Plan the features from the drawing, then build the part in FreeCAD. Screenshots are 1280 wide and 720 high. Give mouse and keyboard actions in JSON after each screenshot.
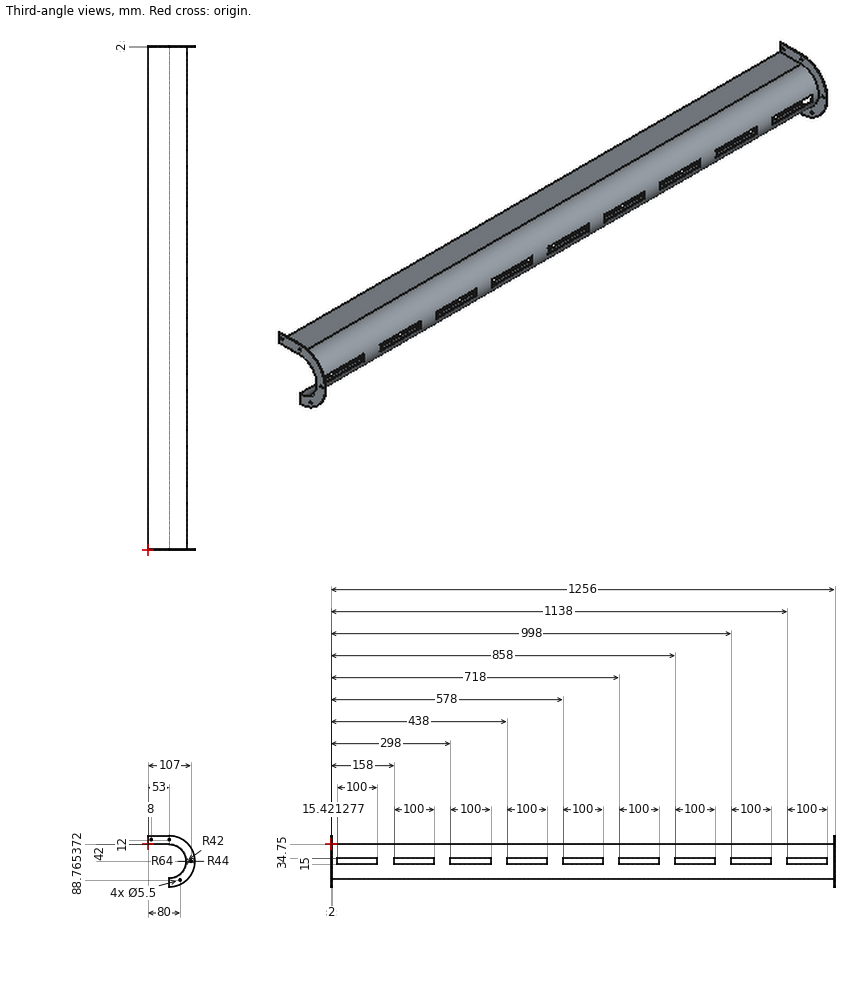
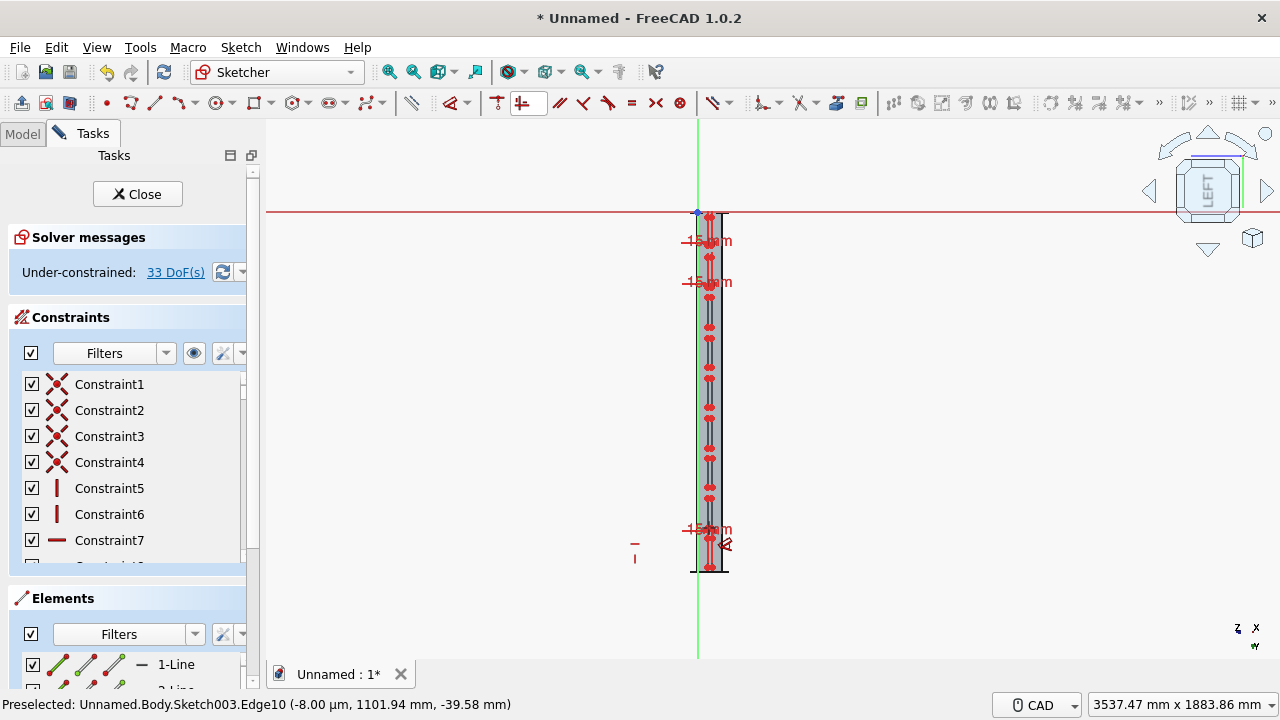
{"action": "scroll", "coordinate": [709, 327], "scroll_direction": "up", "scroll_amount": 12}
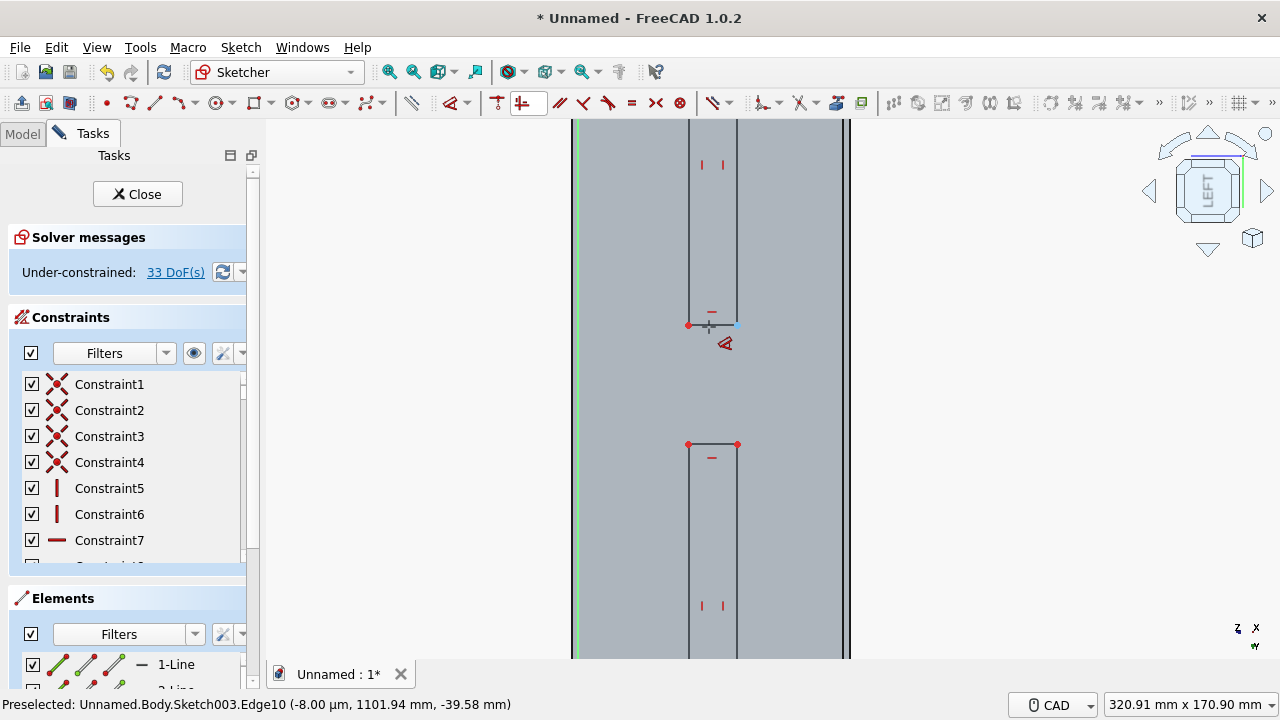
{"action": "left_click", "coordinate": [703, 325]}
{"action": "left_click", "coordinate": [713, 291]}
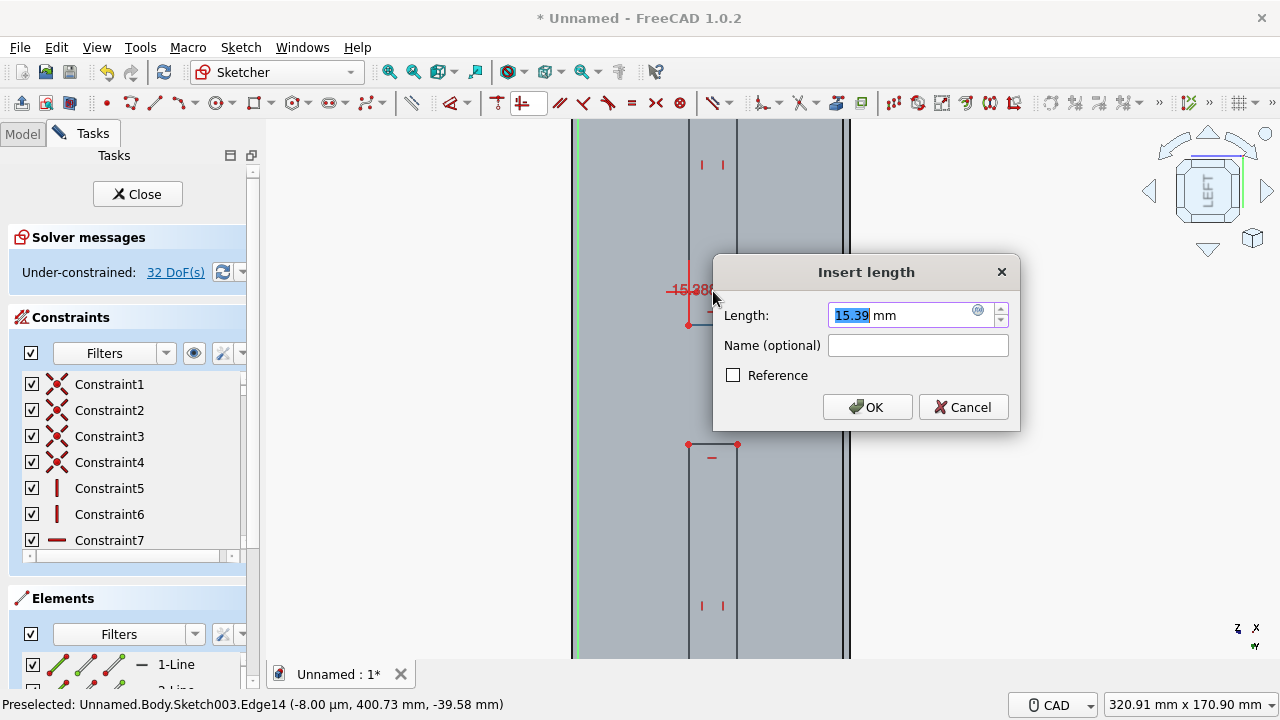
{"action": "type", "text": "15"}
{"action": "key", "text": "Return"}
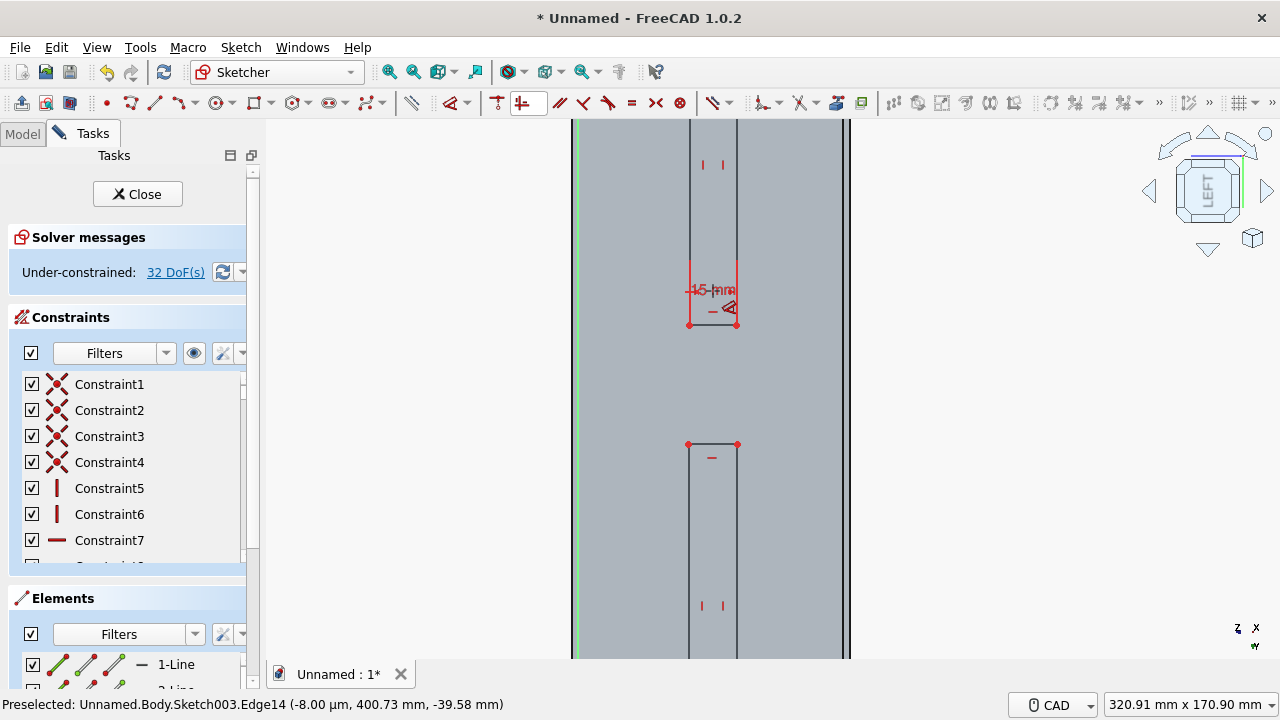
{"action": "scroll", "coordinate": [709, 327], "scroll_direction": "down", "scroll_amount": 12}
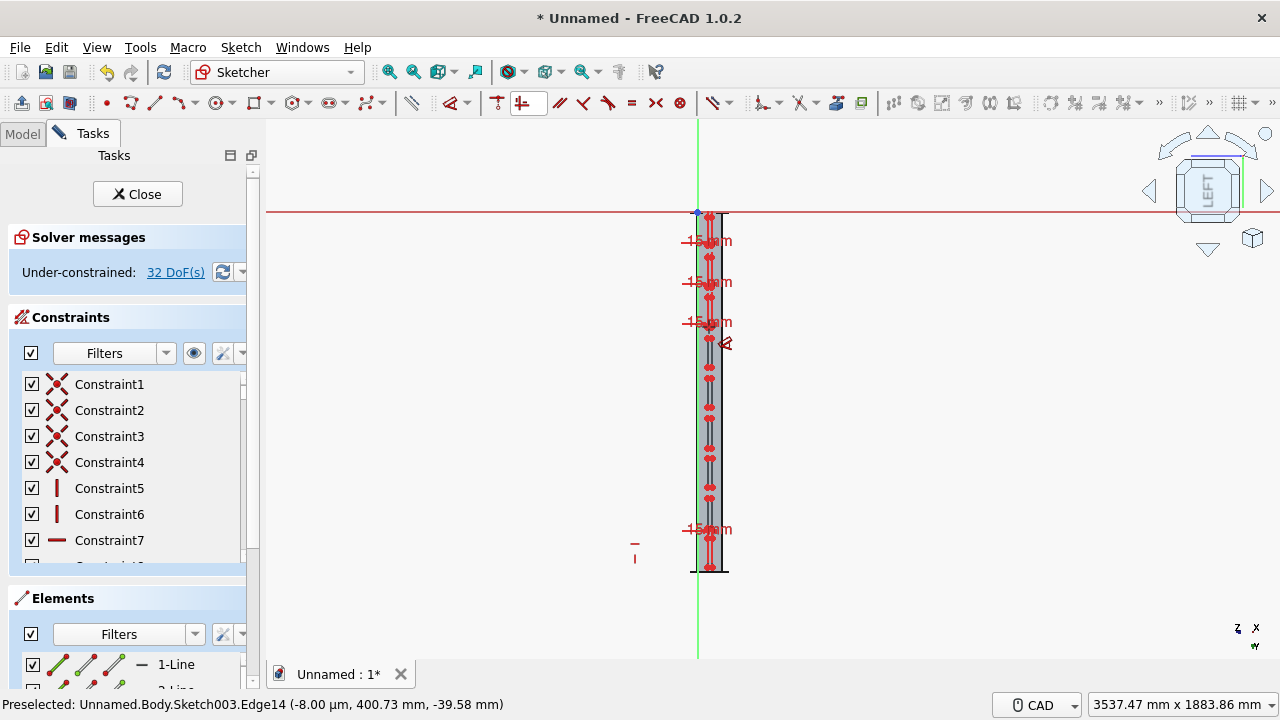
{"action": "scroll", "coordinate": [709, 367], "scroll_direction": "up", "scroll_amount": 12}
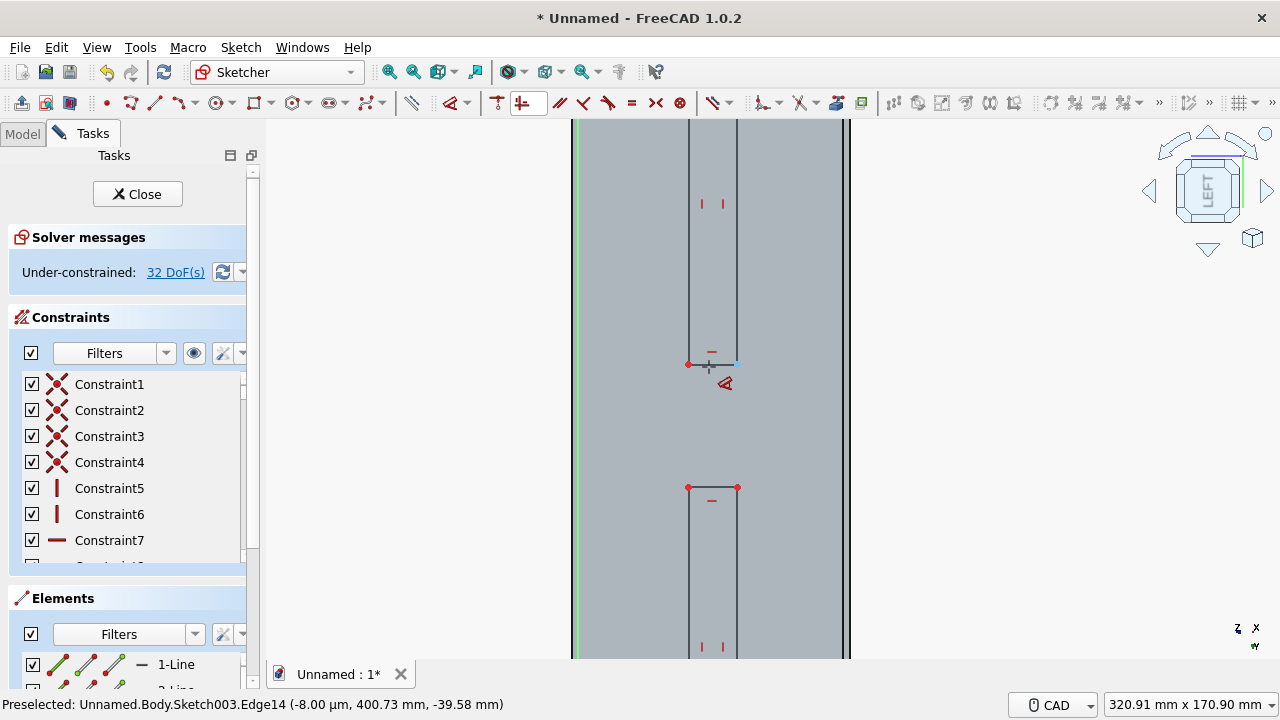
{"action": "left_click", "coordinate": [703, 365]}
{"action": "left_click", "coordinate": [713, 331]}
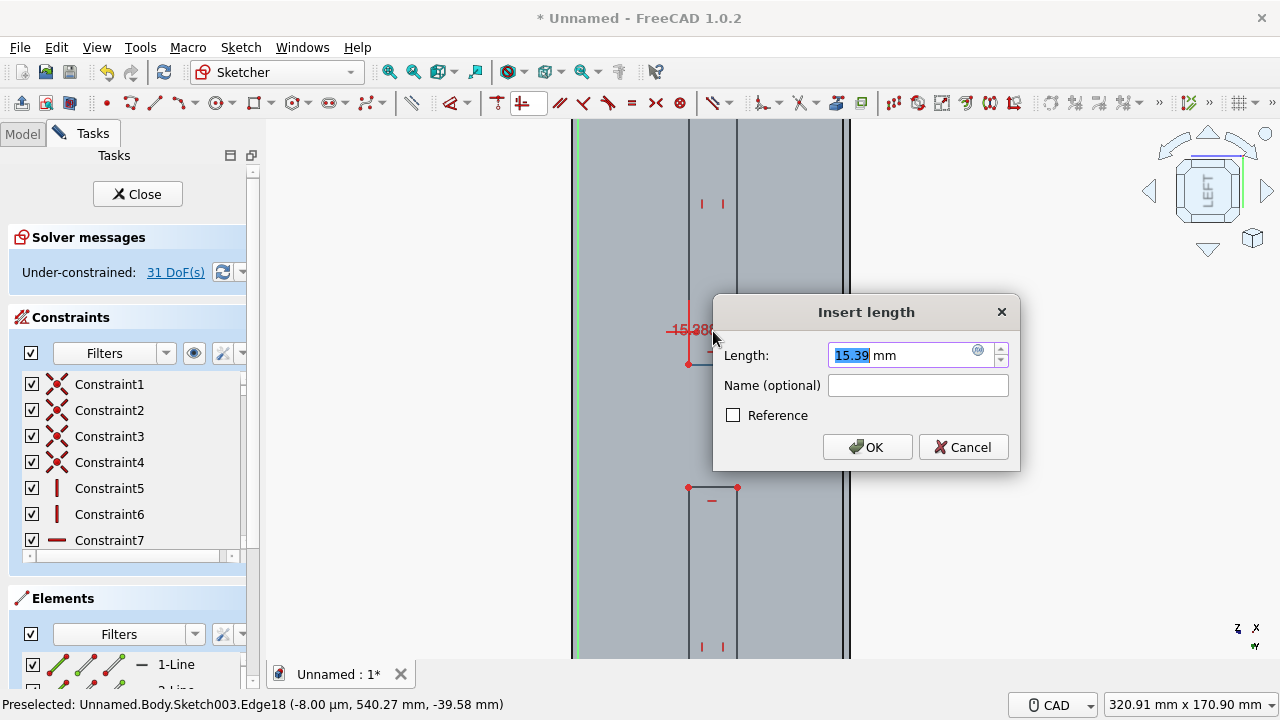
{"action": "type", "text": "15"}
{"action": "key", "text": "Return"}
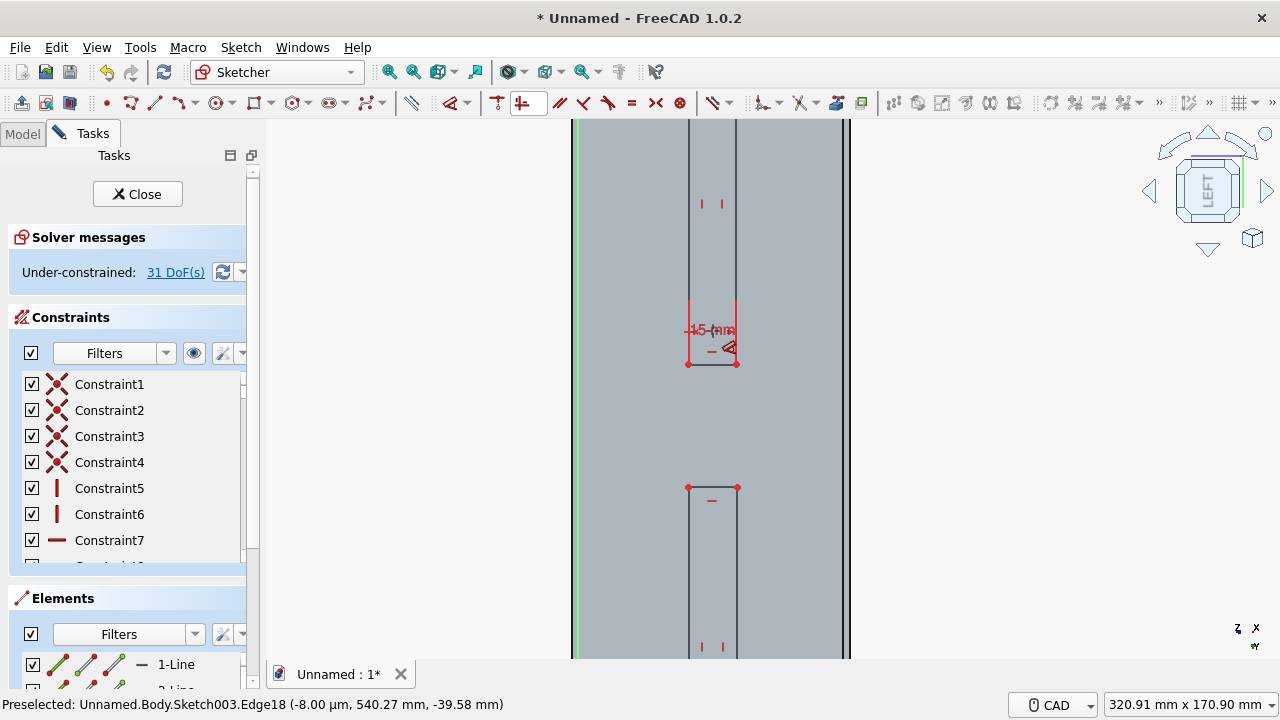
{"action": "scroll", "coordinate": [709, 367], "scroll_direction": "down", "scroll_amount": 12}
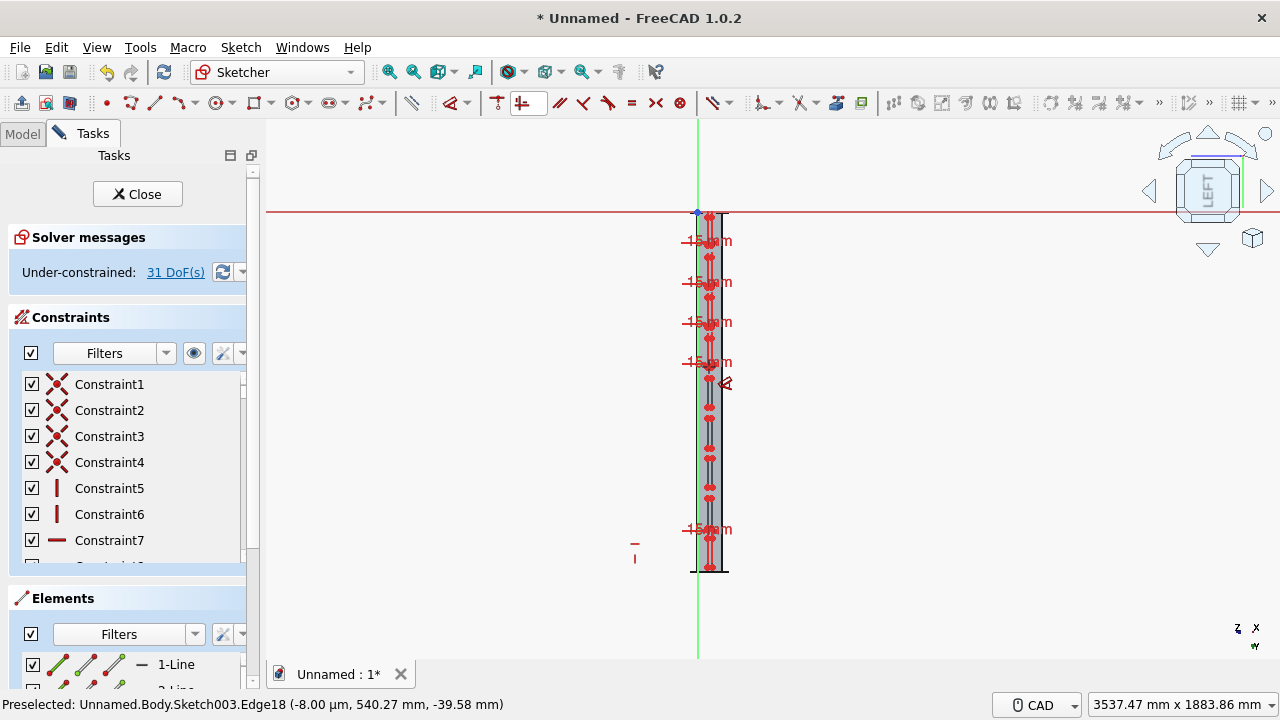
{"action": "scroll", "coordinate": [709, 407], "scroll_direction": "up", "scroll_amount": 12}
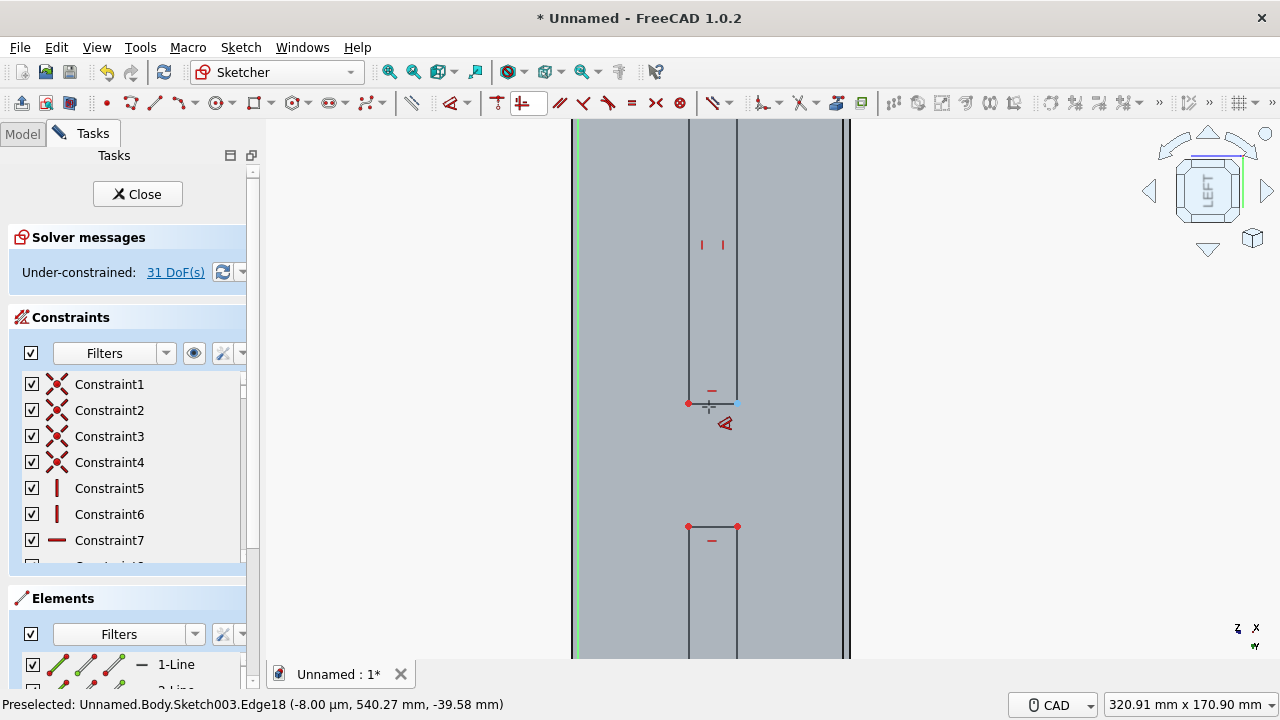
{"action": "left_click", "coordinate": [703, 404]}
{"action": "left_click", "coordinate": [713, 438]}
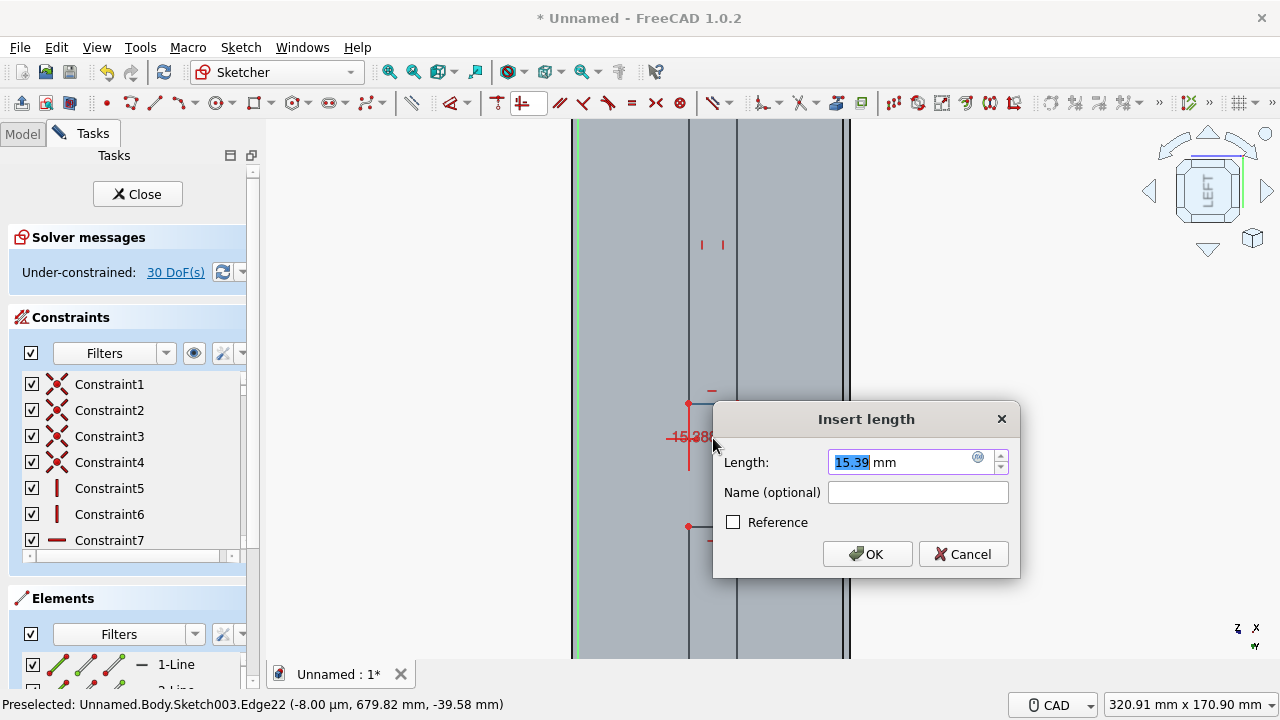
{"action": "type", "text": "15"}
{"action": "key", "text": "Return"}